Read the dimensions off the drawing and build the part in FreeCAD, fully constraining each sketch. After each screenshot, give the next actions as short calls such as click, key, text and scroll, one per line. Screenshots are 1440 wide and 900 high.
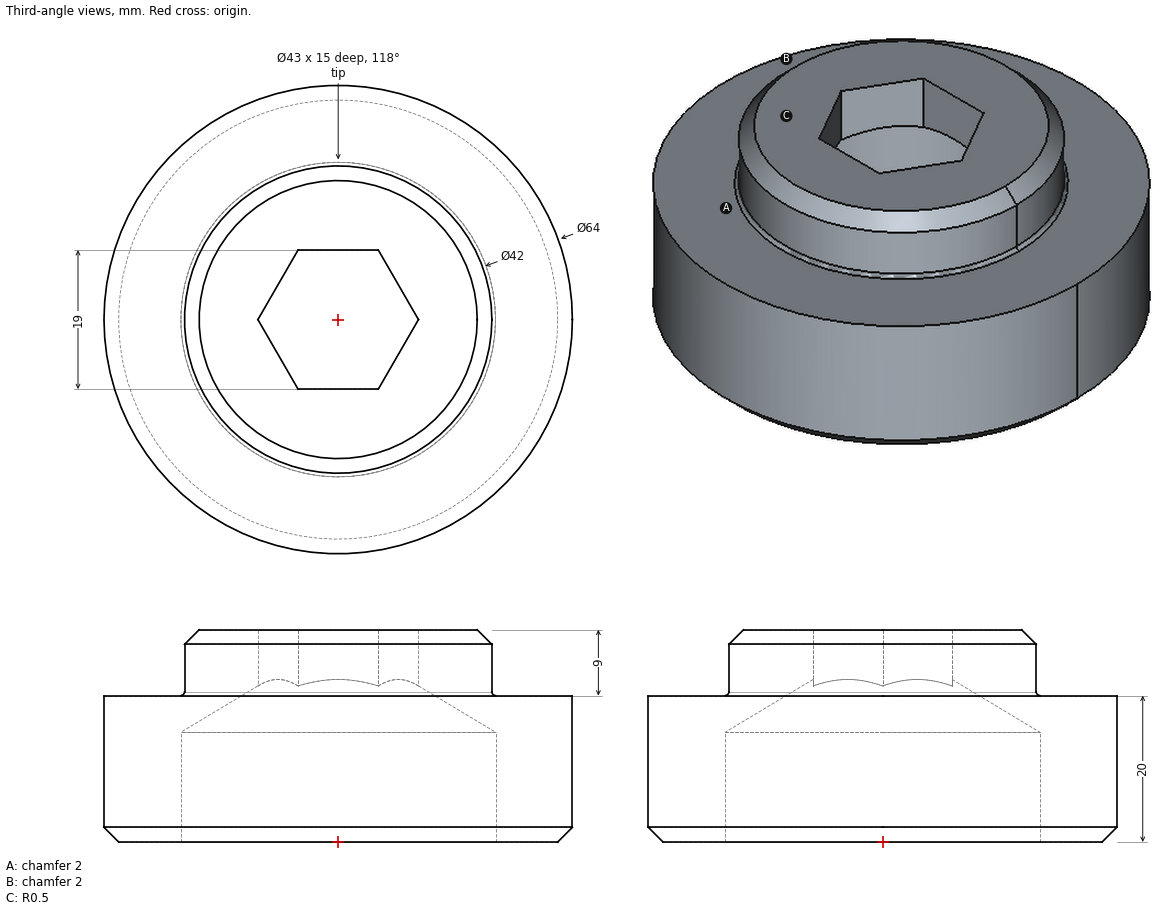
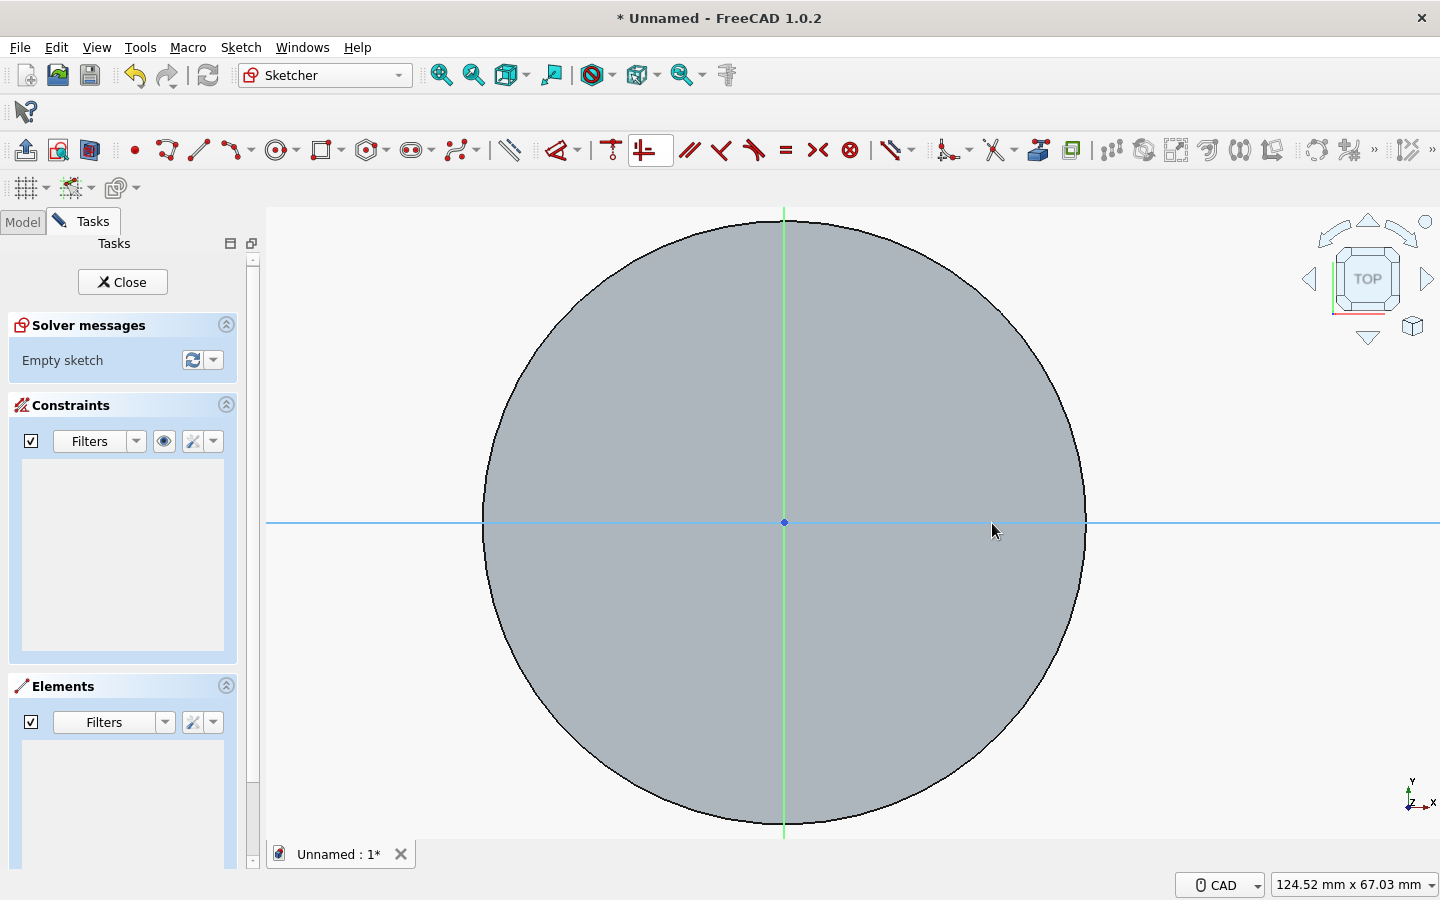
click(276, 150)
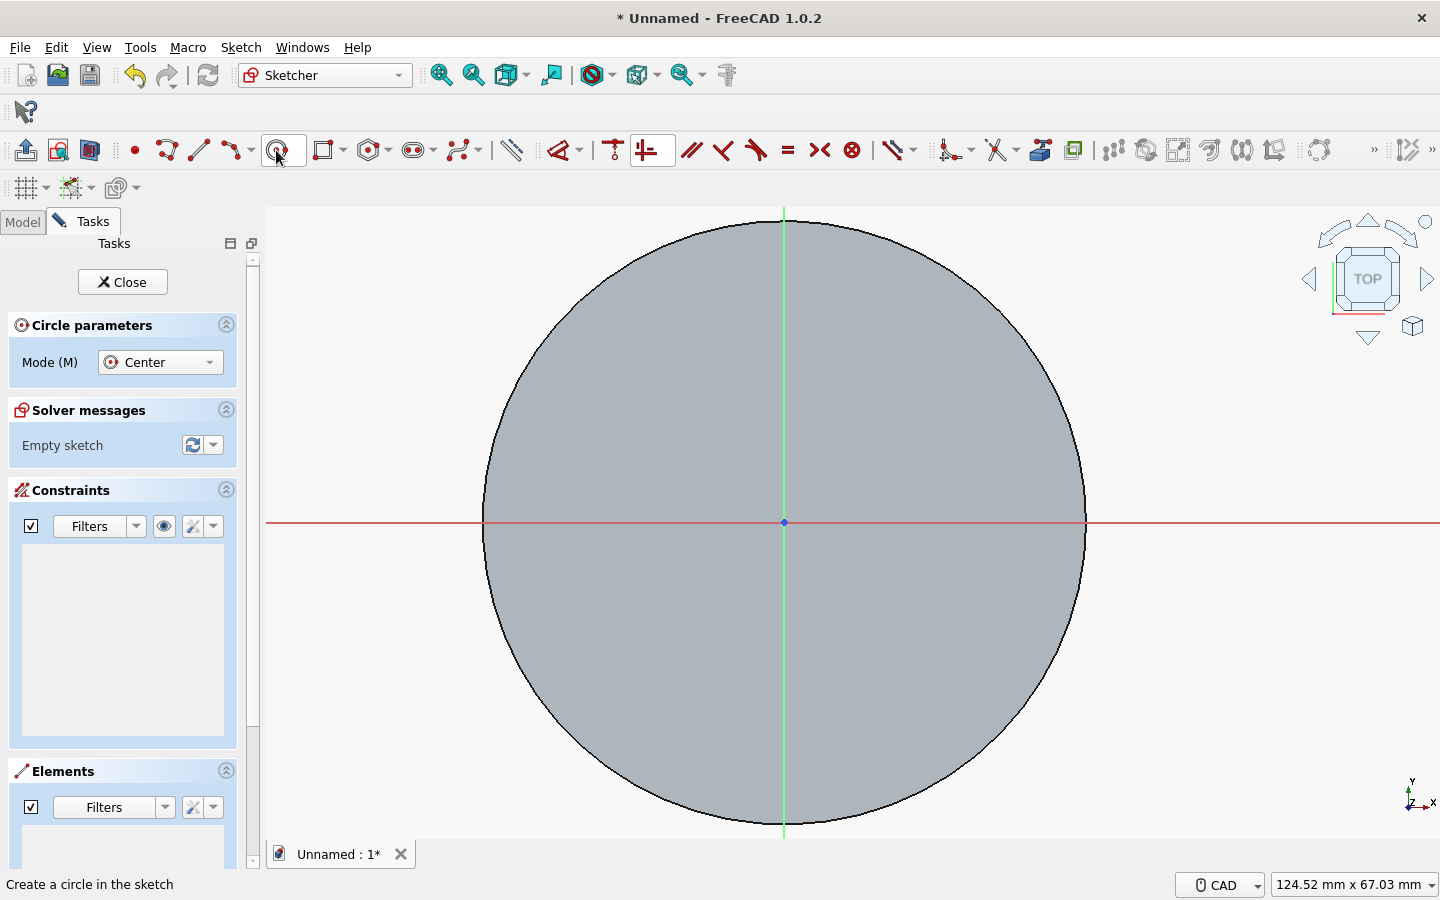
click(784, 523)
move(924, 383)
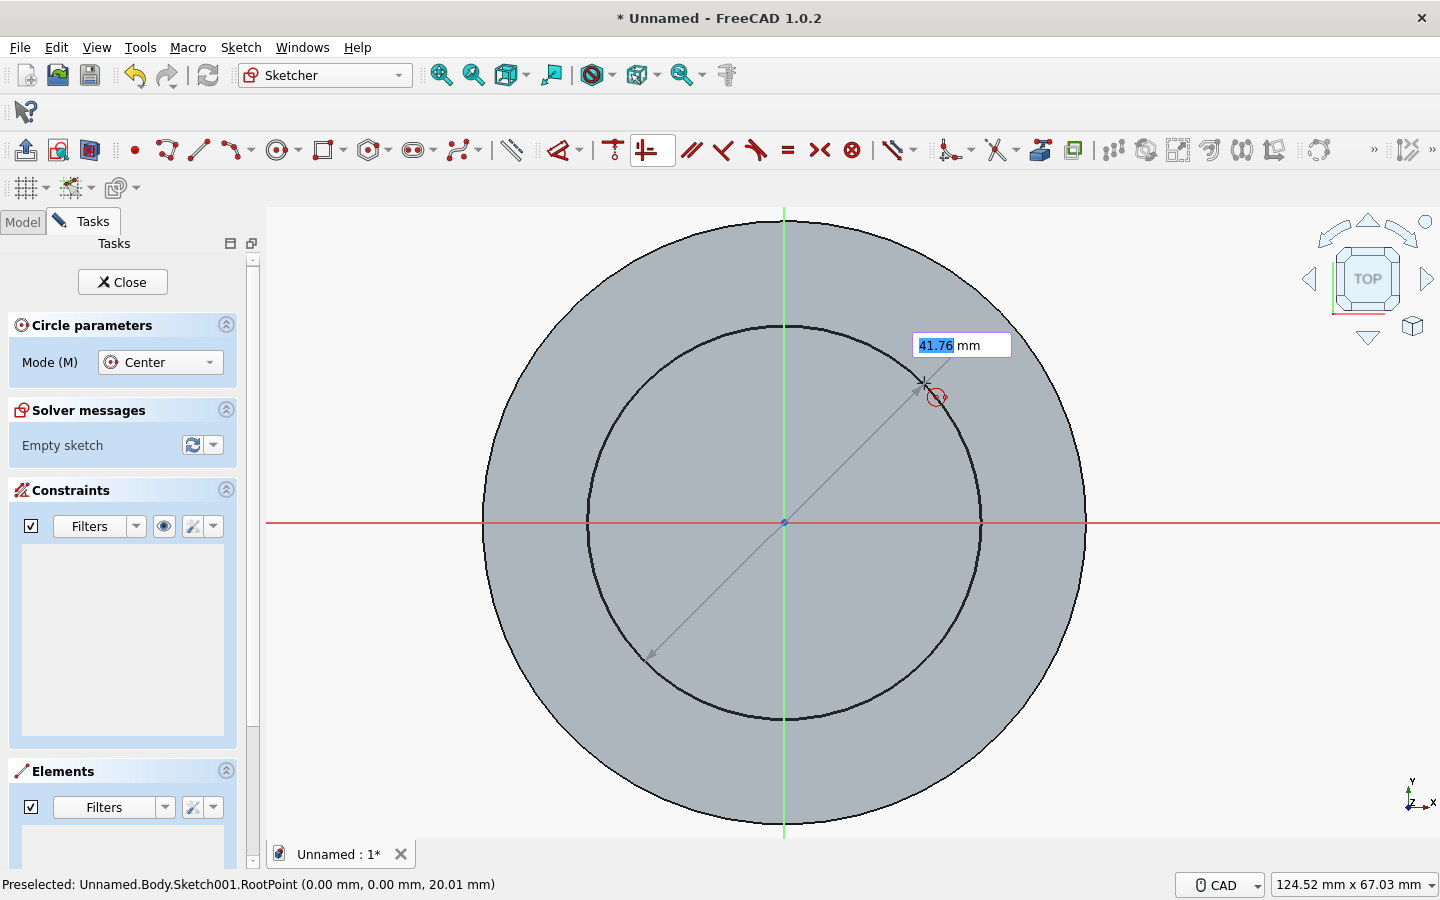
text(42)
key(Return)
key(Escape)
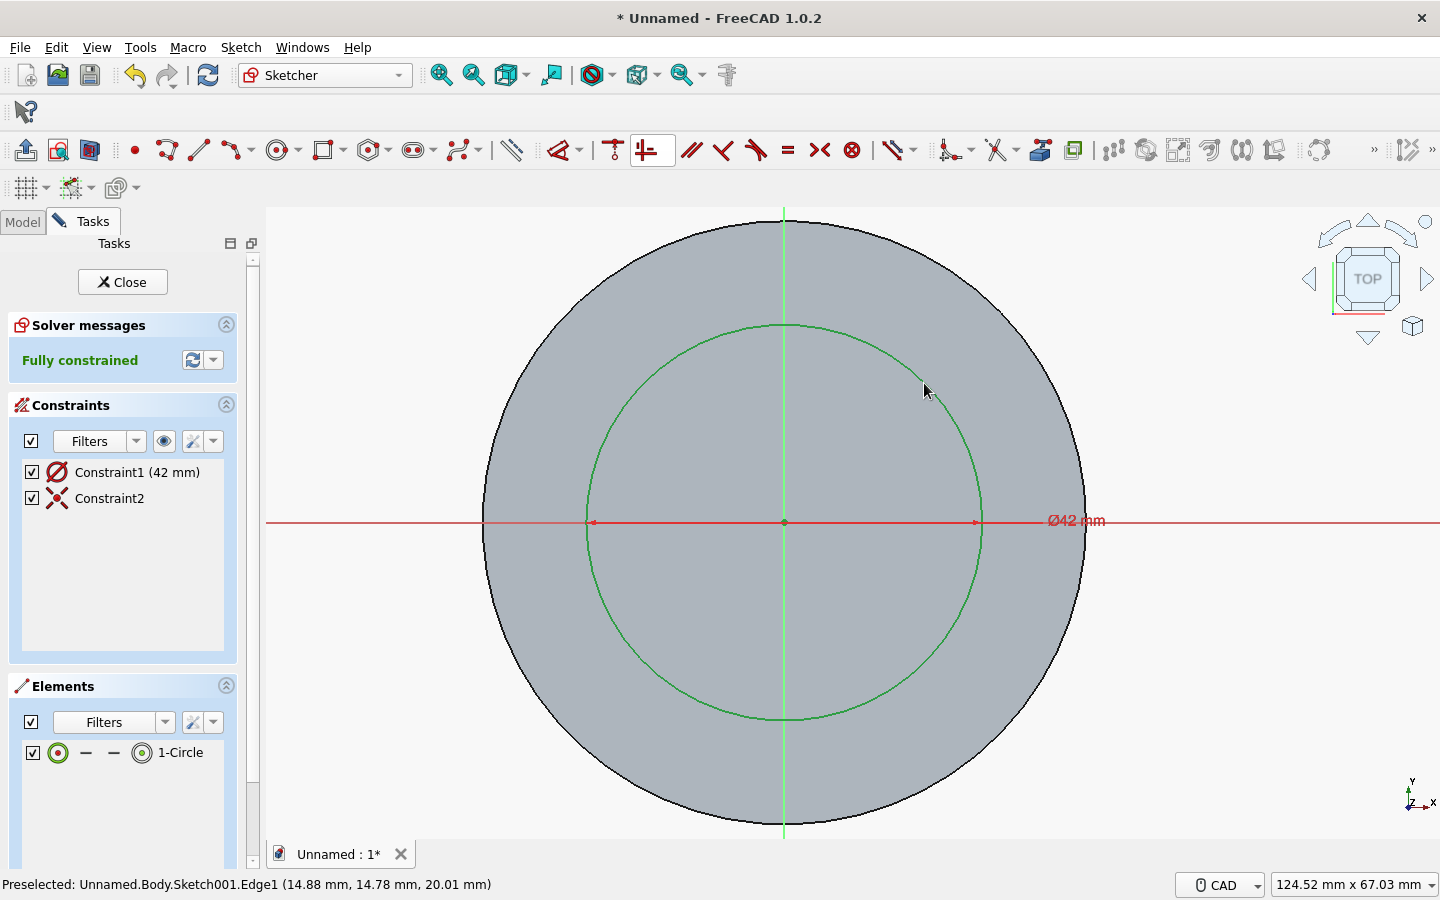
click(123, 282)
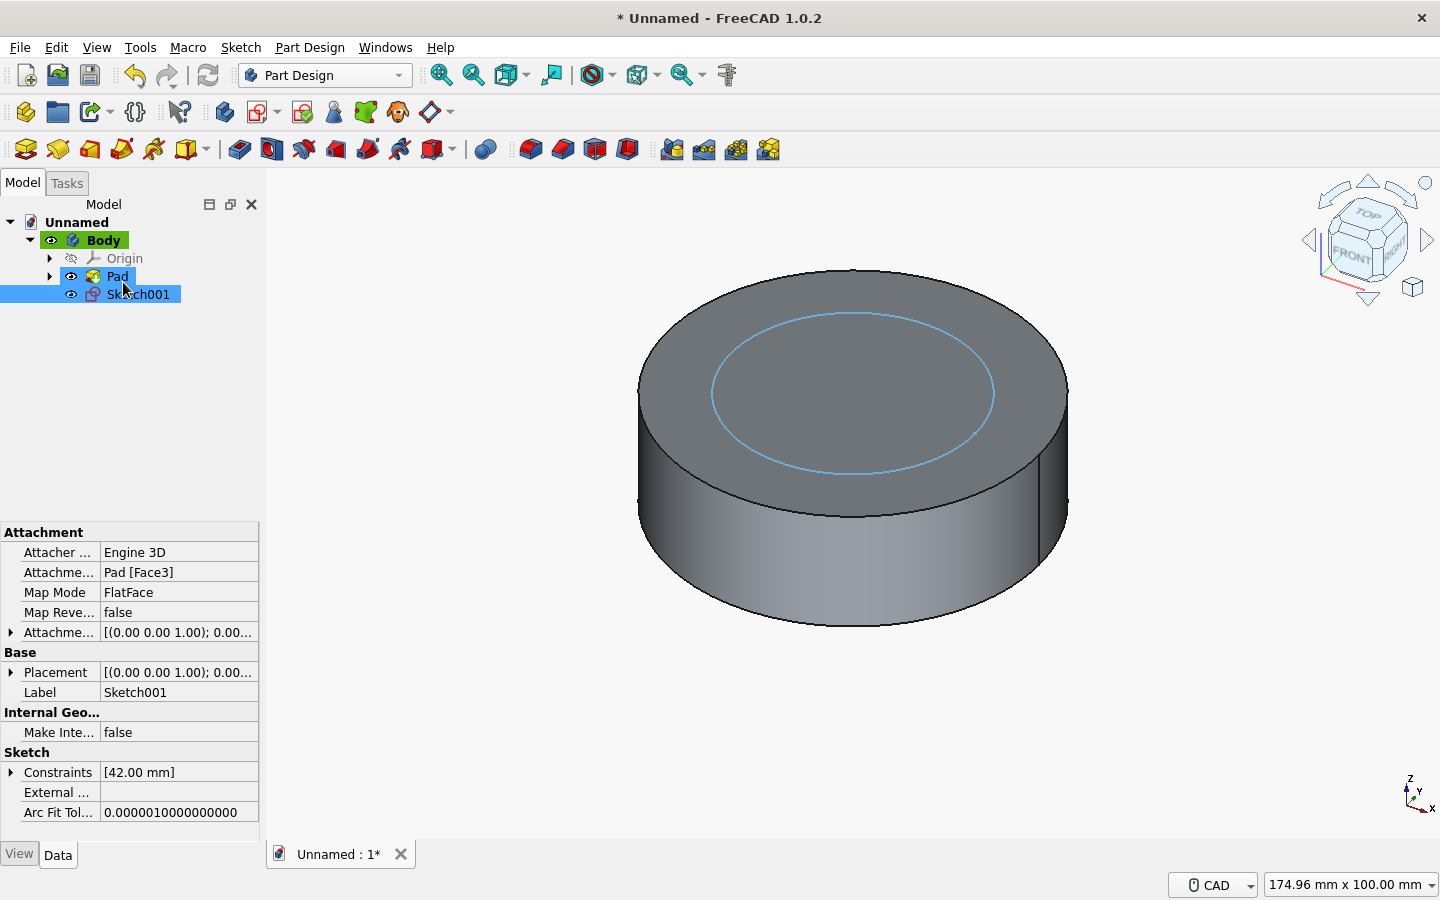
click(26, 150)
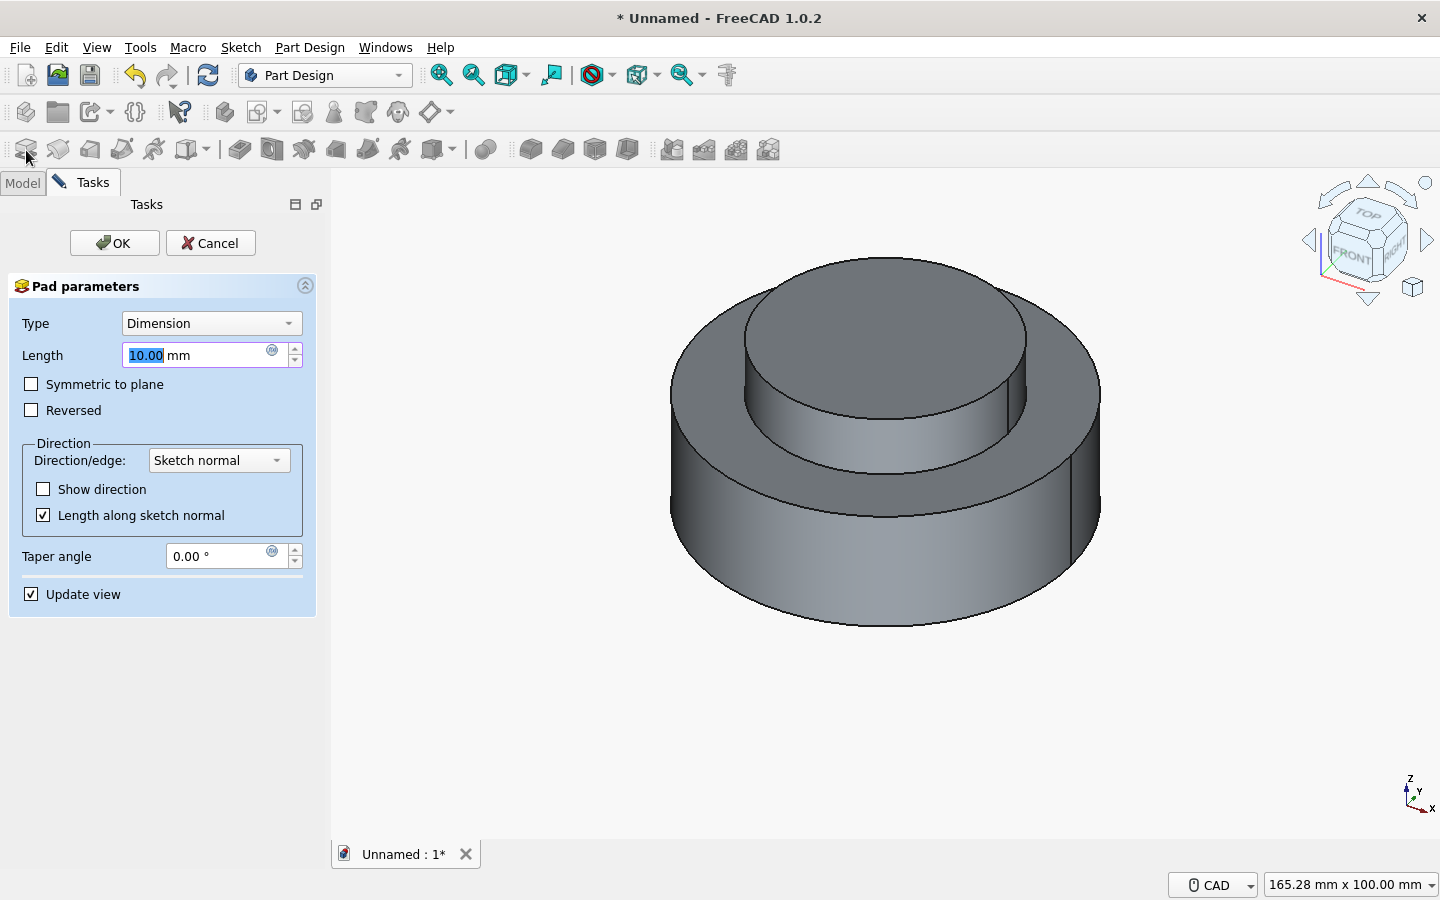
text(9)
key(Tab)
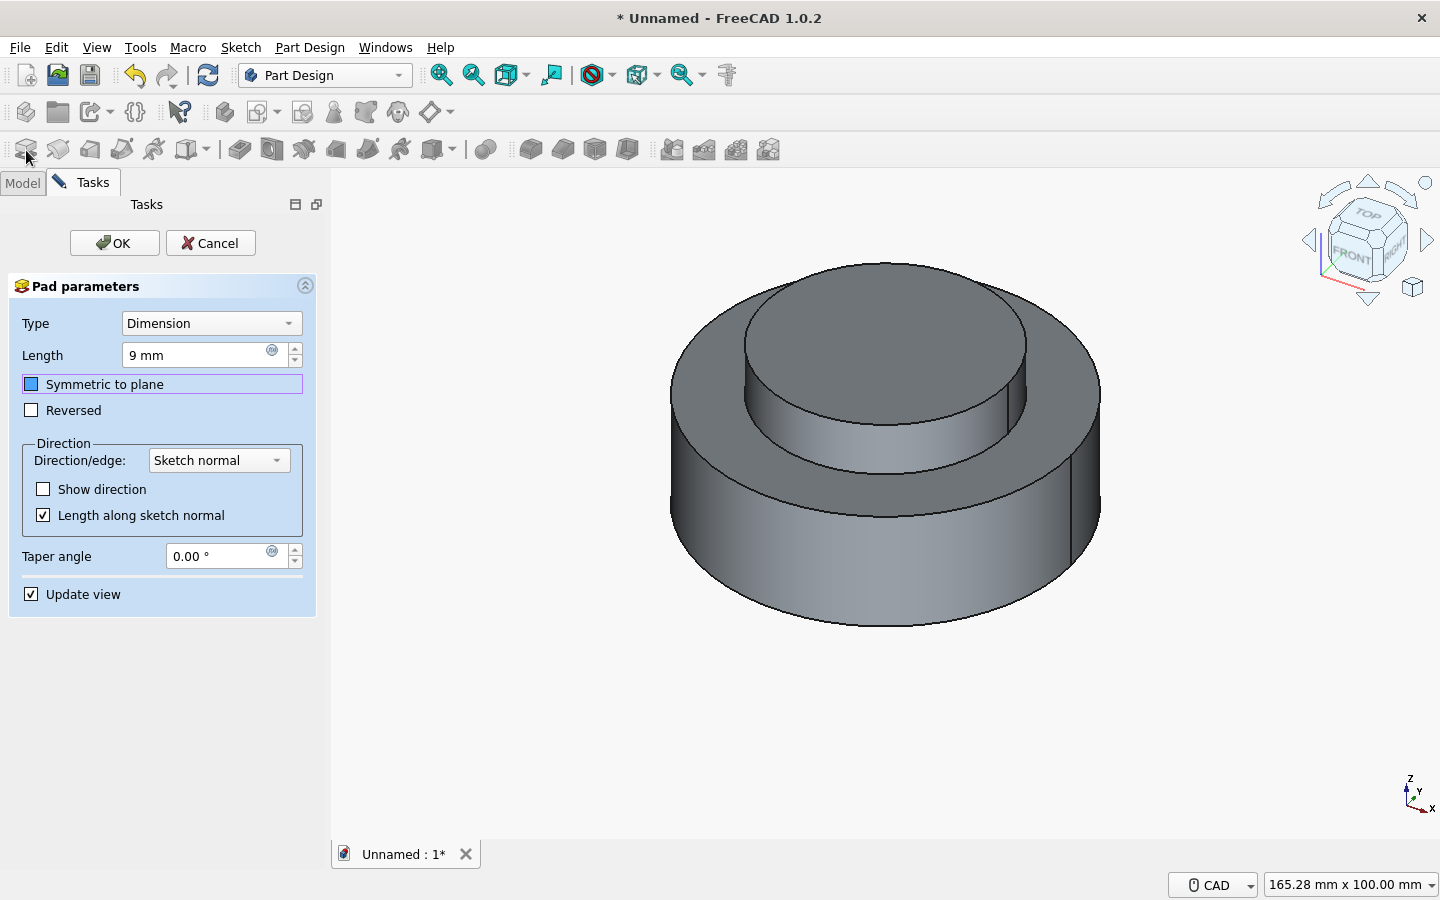
click(115, 243)